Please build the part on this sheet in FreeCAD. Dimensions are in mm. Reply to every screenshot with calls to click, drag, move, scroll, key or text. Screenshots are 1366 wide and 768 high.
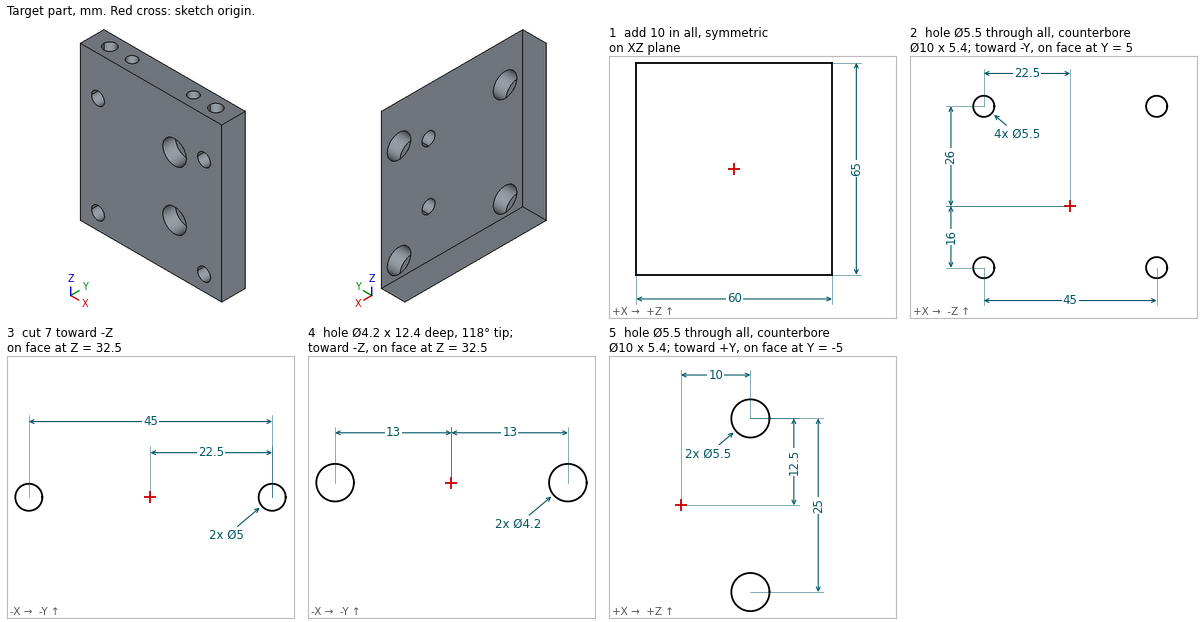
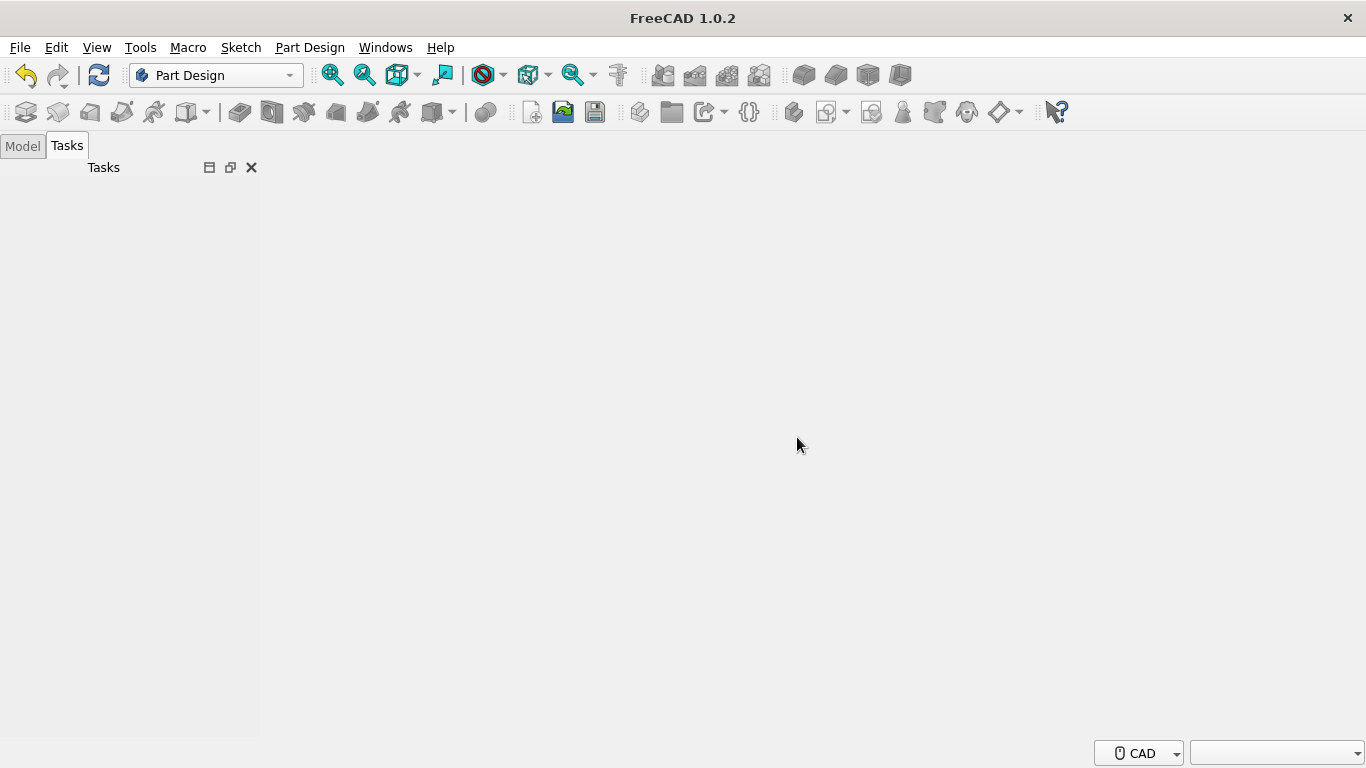
key(ctrl+n)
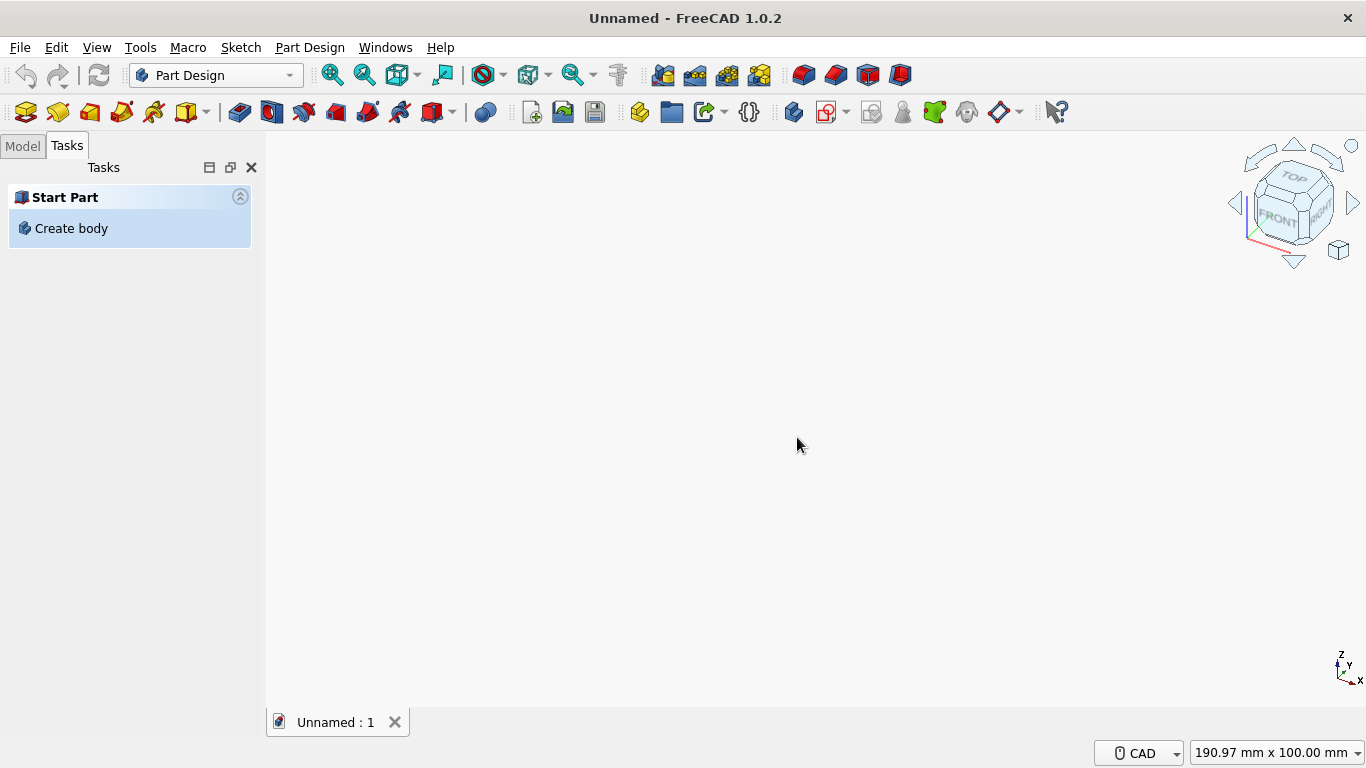
click(826, 112)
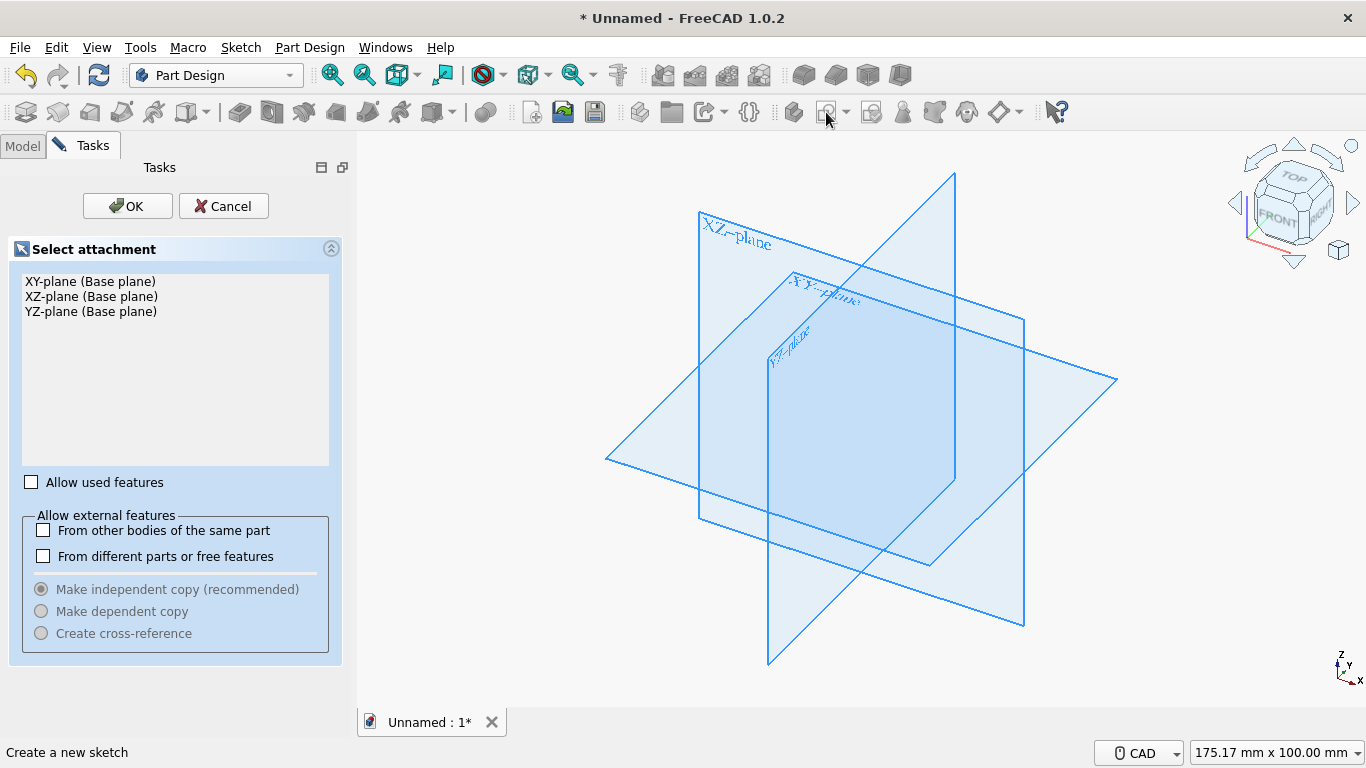
click(82, 296)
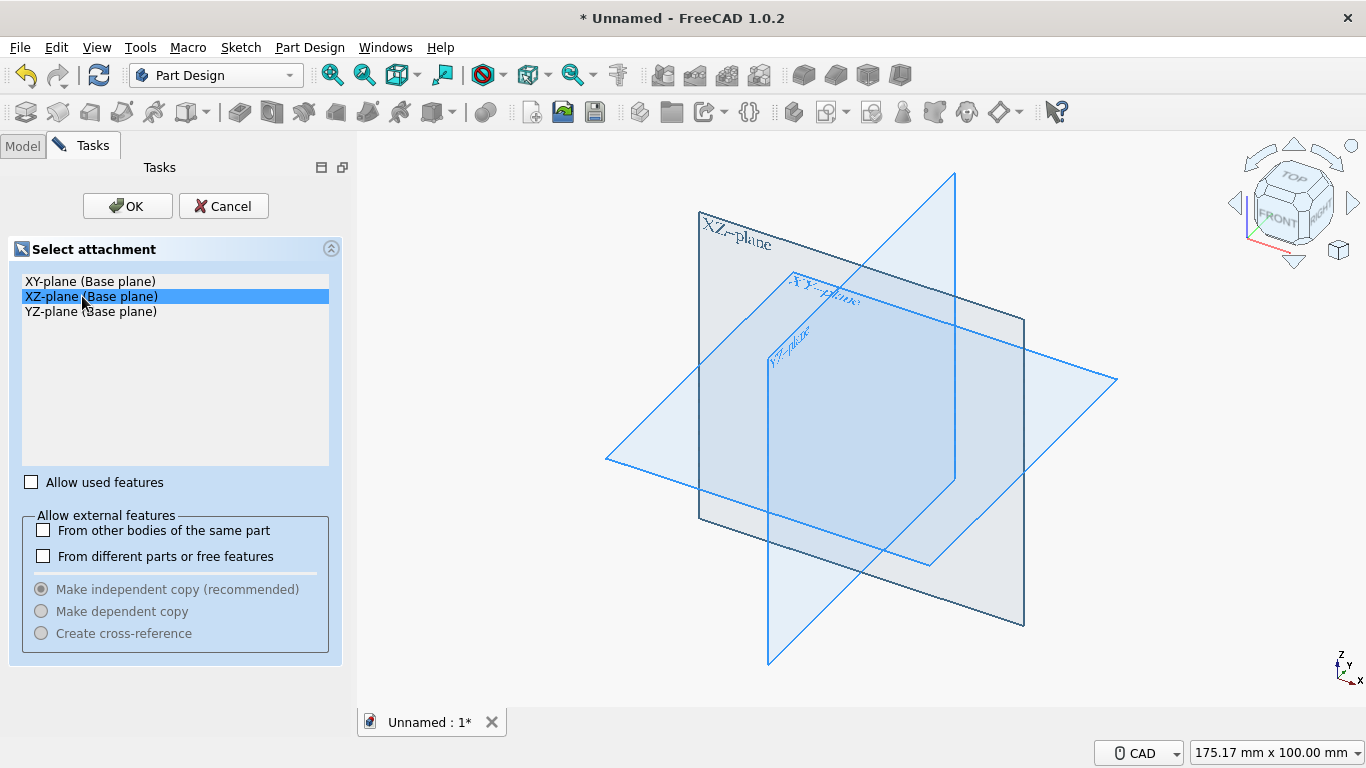
click(128, 206)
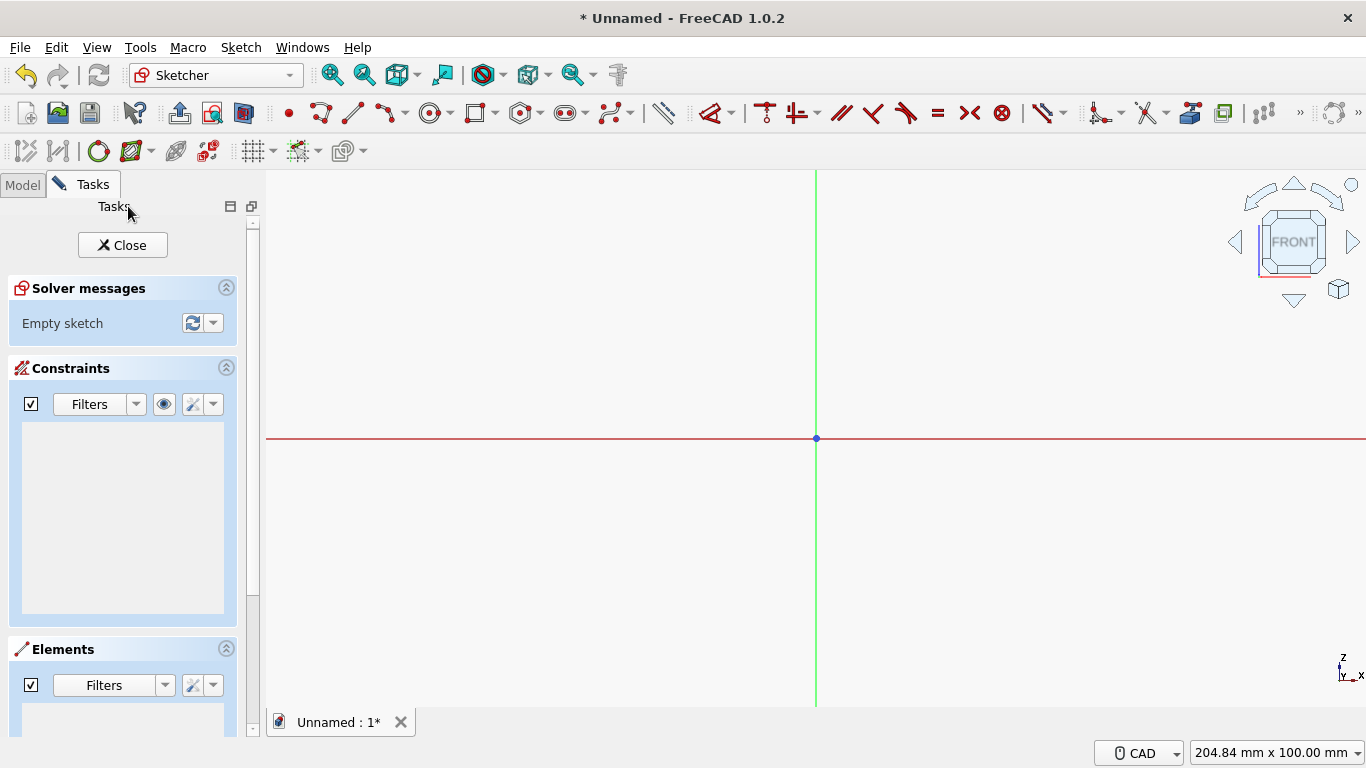
key(g)
key(v)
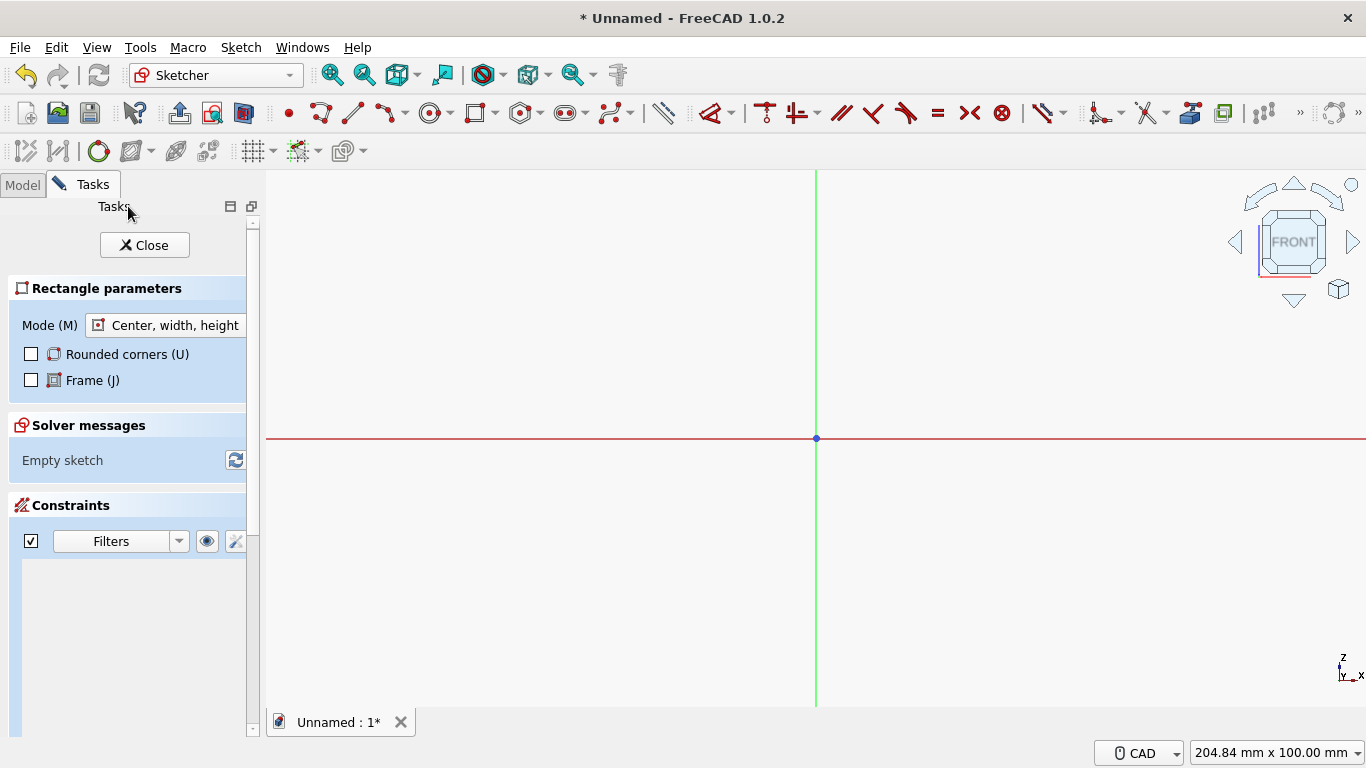
click(816, 438)
click(977, 264)
key(Escape)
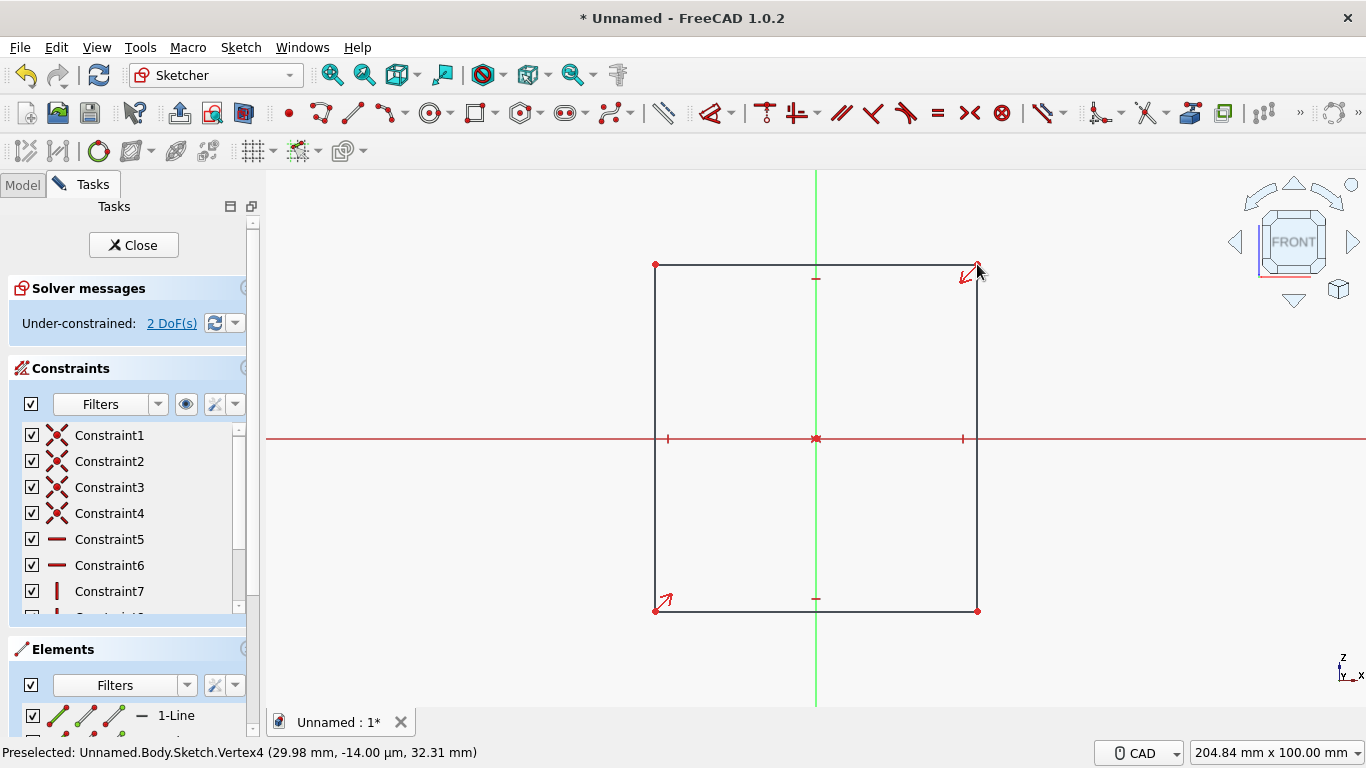
click(752, 612)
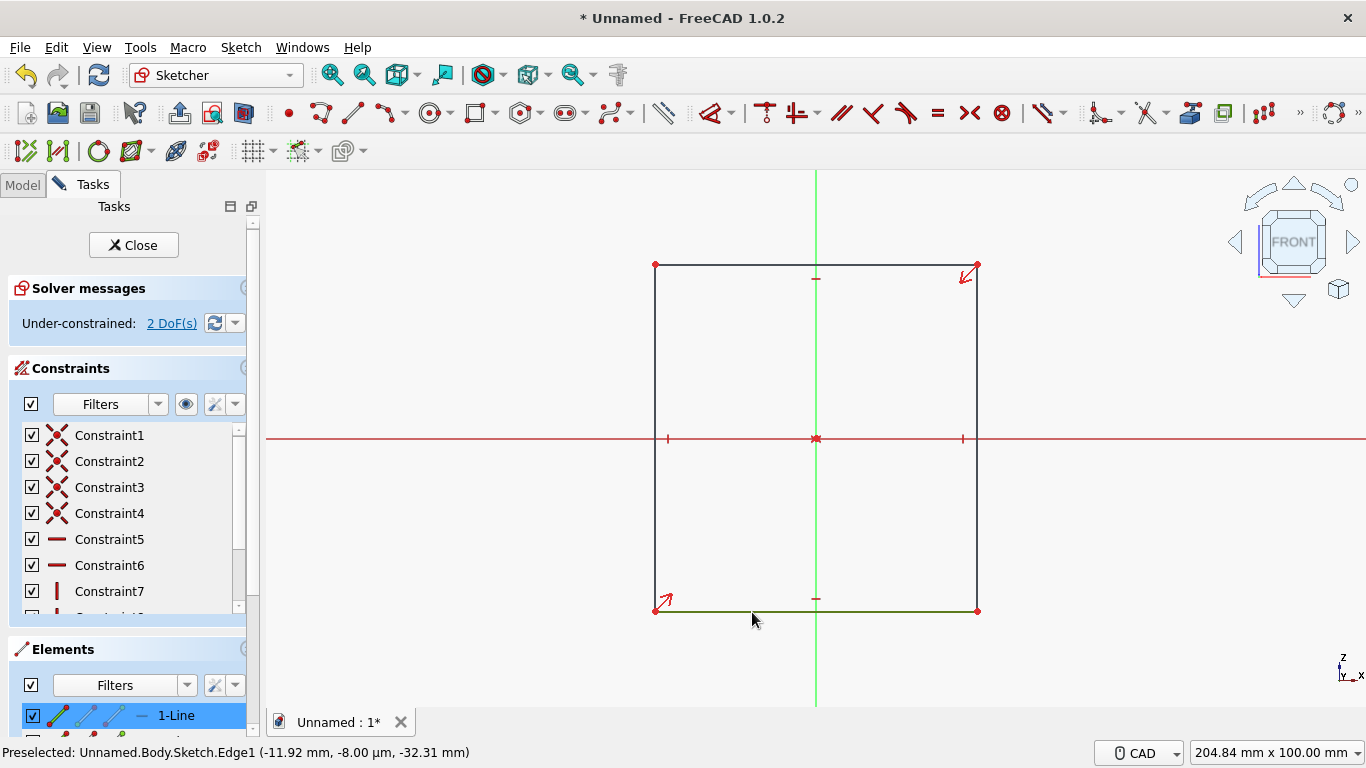
key(l)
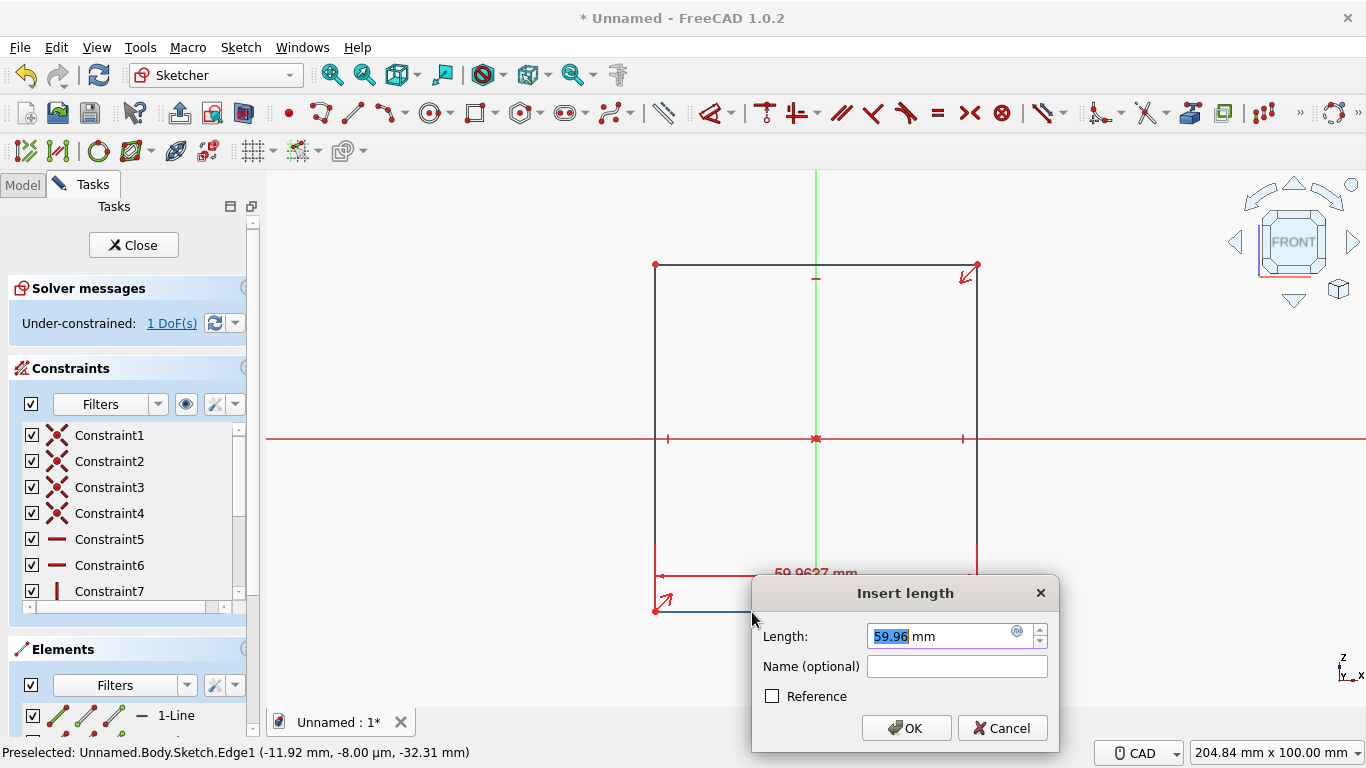
text(60)
key(Return)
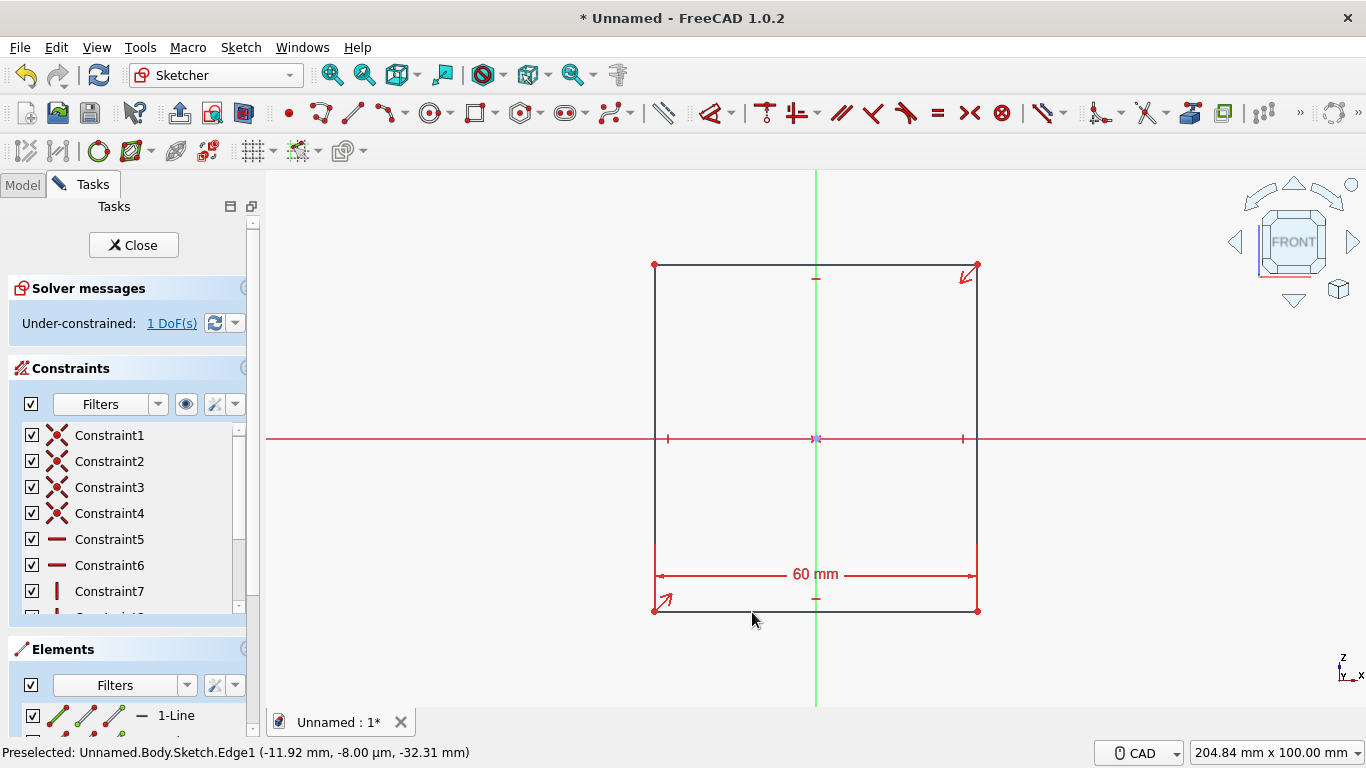
click(977, 508)